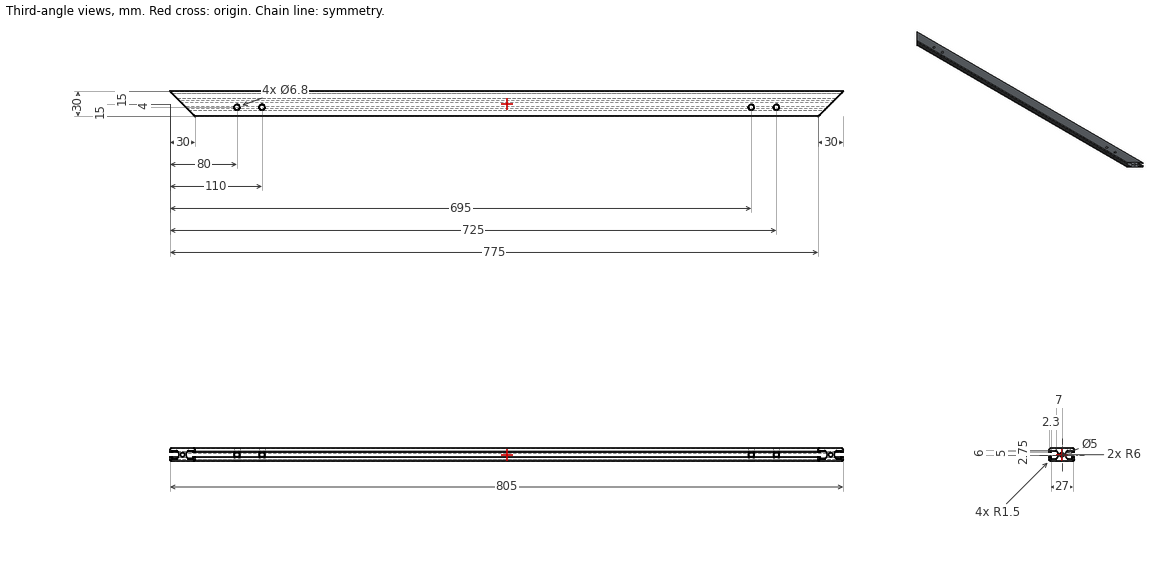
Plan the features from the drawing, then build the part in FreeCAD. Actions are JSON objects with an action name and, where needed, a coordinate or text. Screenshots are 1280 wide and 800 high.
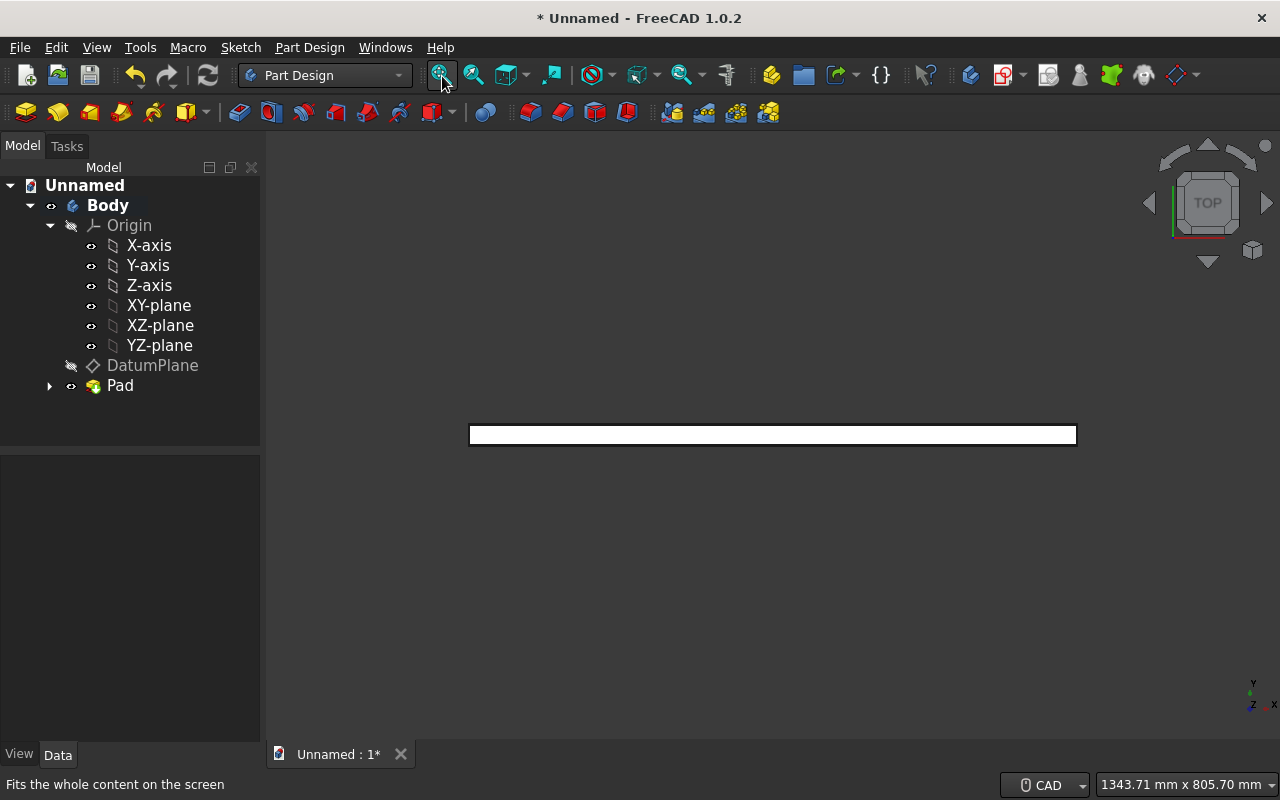
{"action": "left_click", "coordinate": [773, 434]}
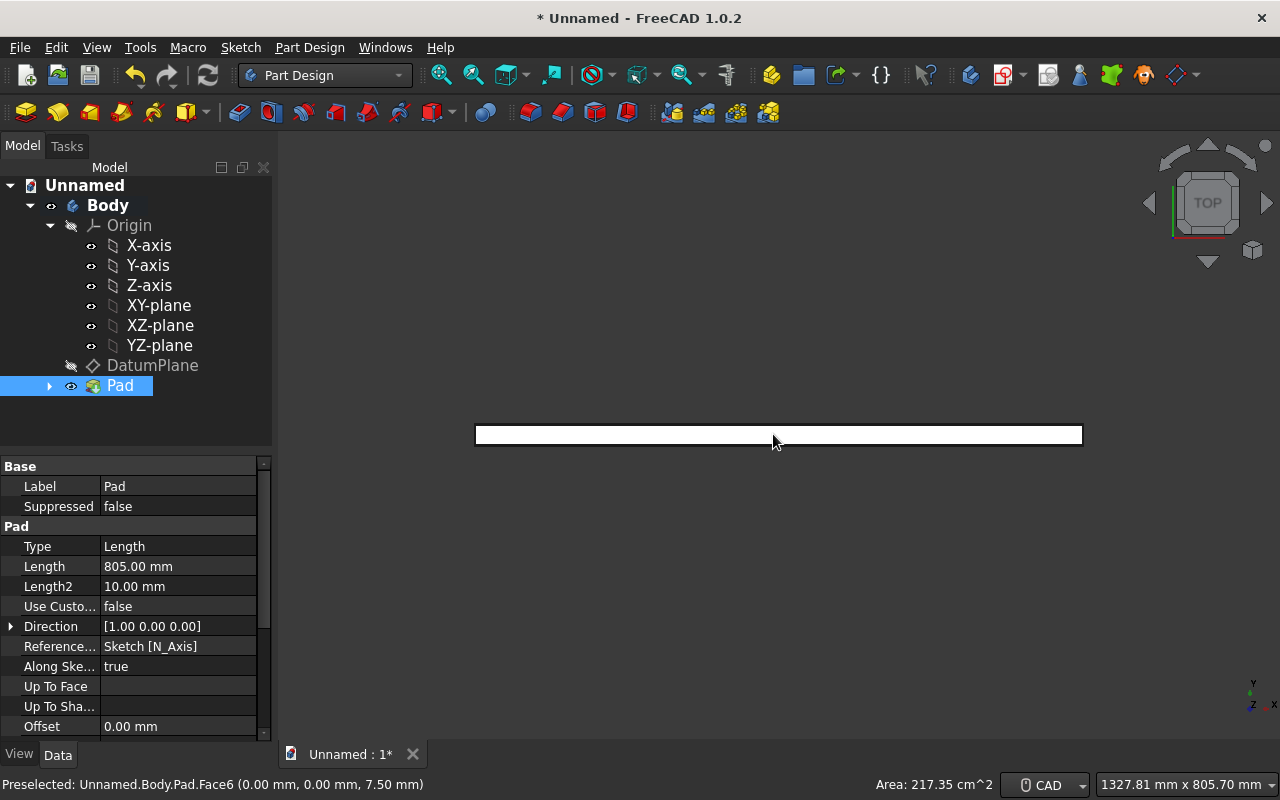
{"action": "left_click", "coordinate": [1004, 76]}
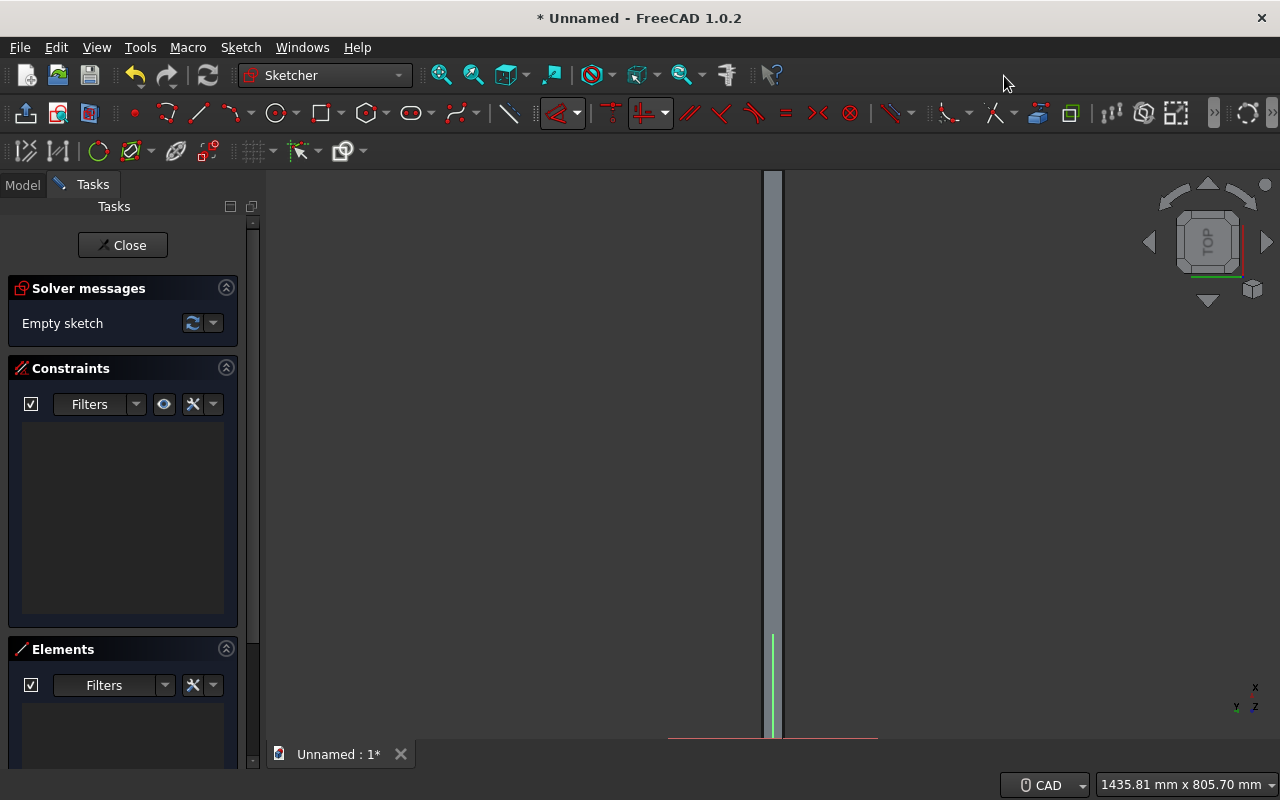
{"action": "scroll", "coordinate": [565, 455], "scroll_direction": "down", "scroll_amount": 2}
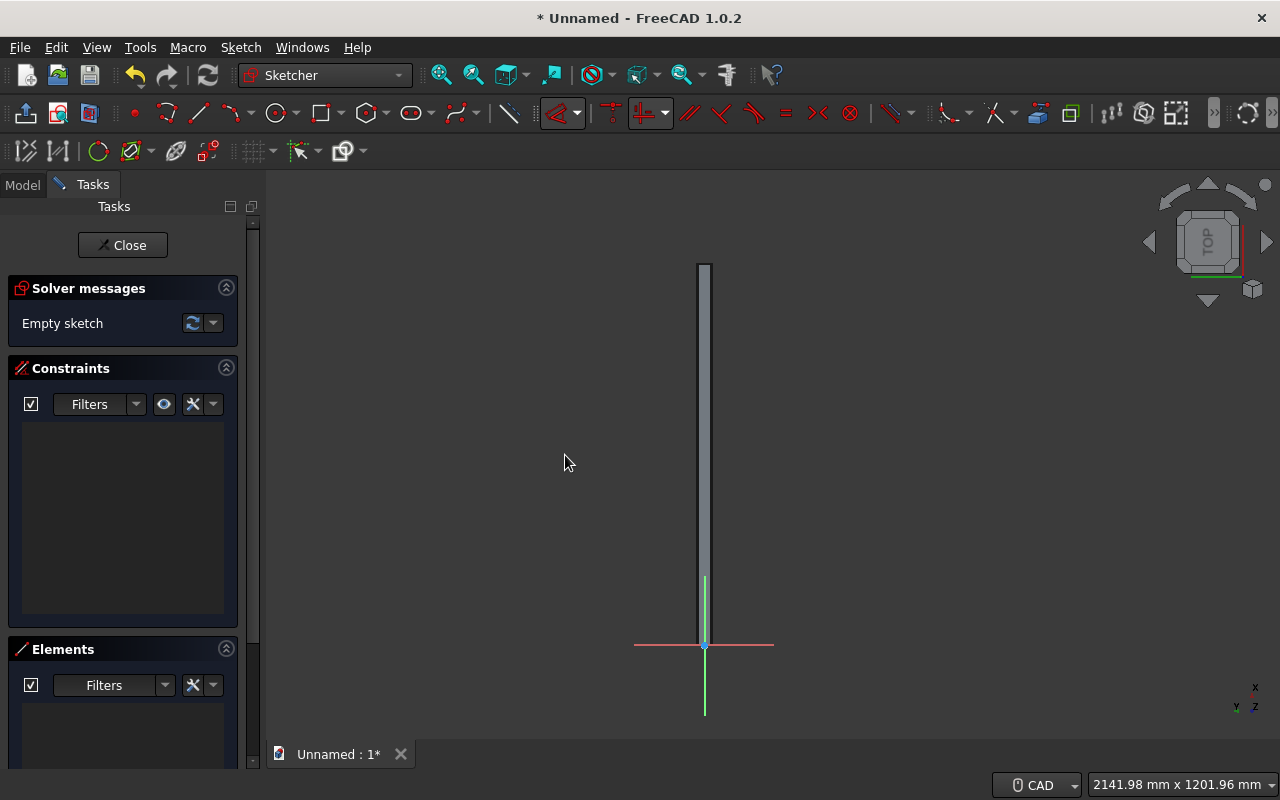
{"action": "left_click", "coordinate": [168, 114]}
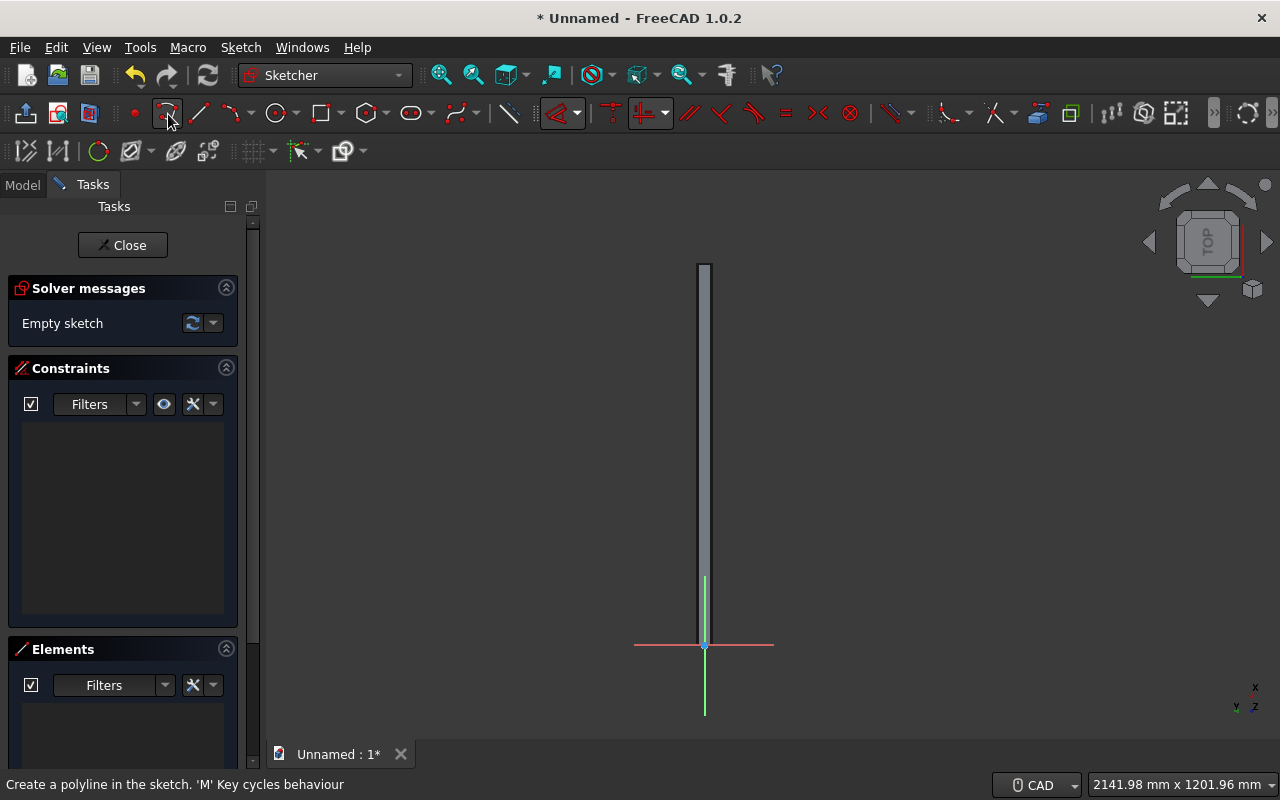
{"action": "scroll", "coordinate": [697, 645], "scroll_direction": "up", "scroll_amount": 5}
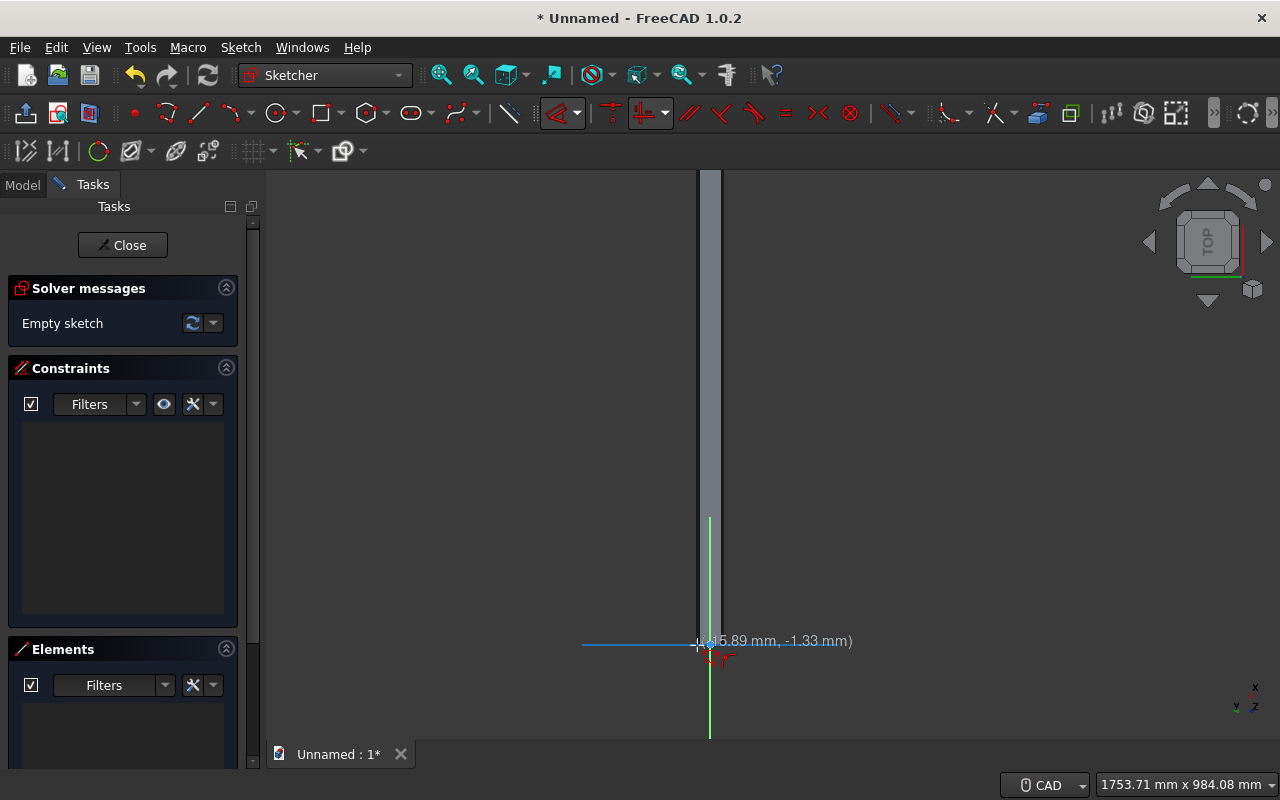
{"action": "left_click", "coordinate": [697, 645]}
{"action": "left_click", "coordinate": [736, 636]}
{"action": "left_click", "coordinate": [736, 606]}
{"action": "left_click", "coordinate": [697, 645]}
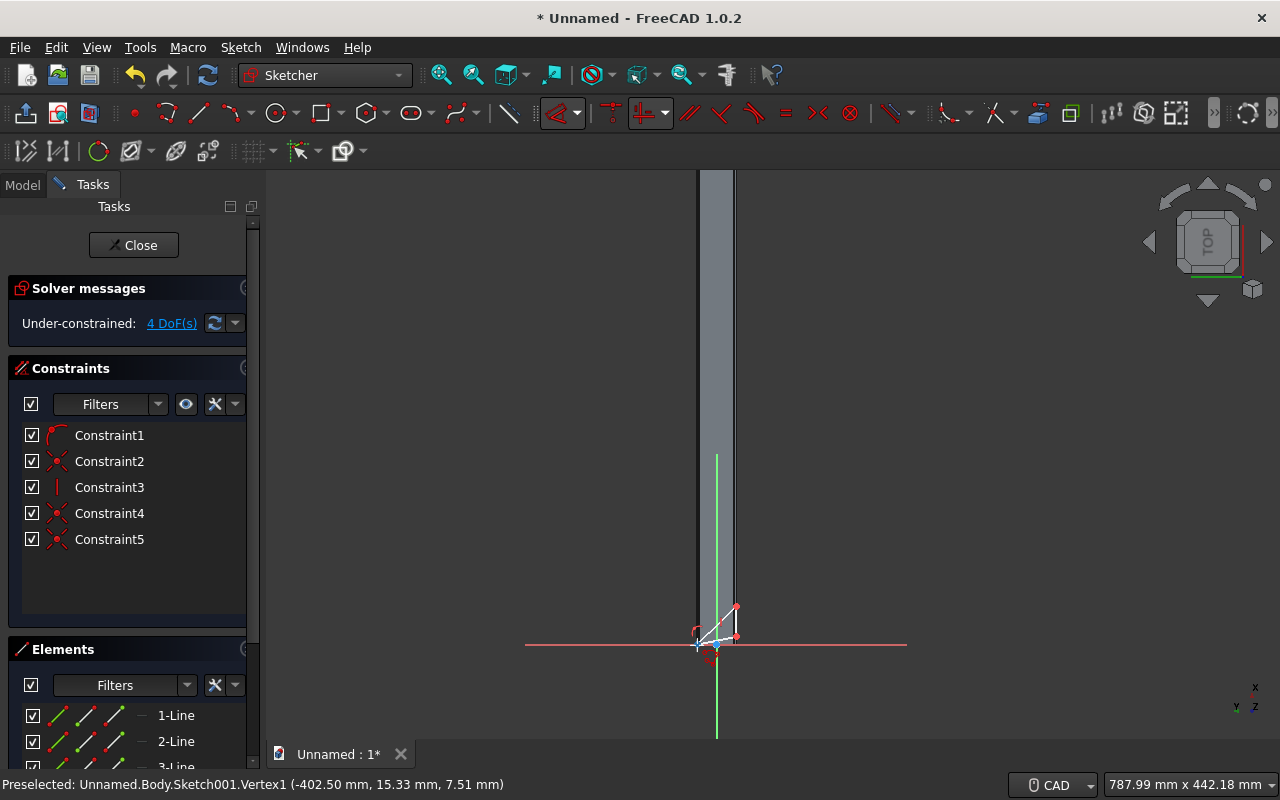
{"action": "scroll", "coordinate": [697, 645], "scroll_direction": "down", "scroll_amount": 5}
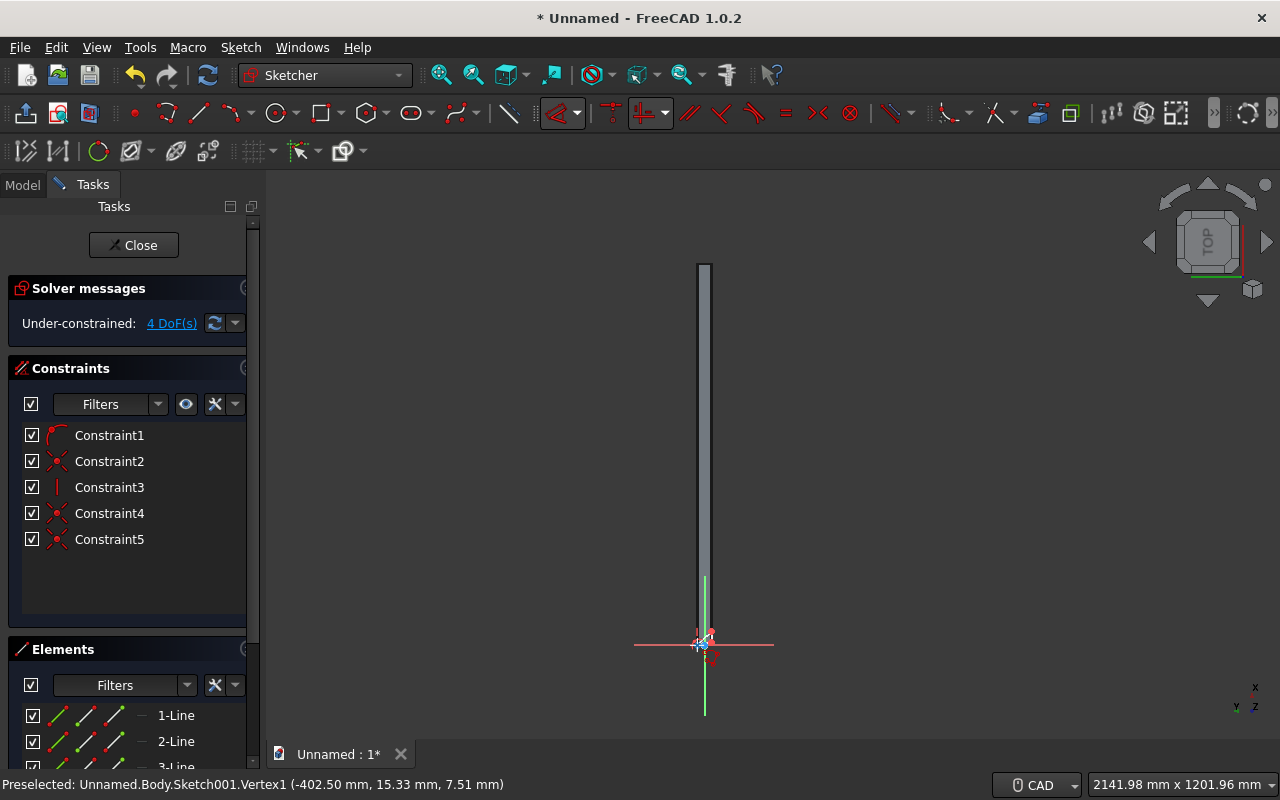
{"action": "scroll", "coordinate": [712, 278], "scroll_direction": "up", "scroll_amount": 5}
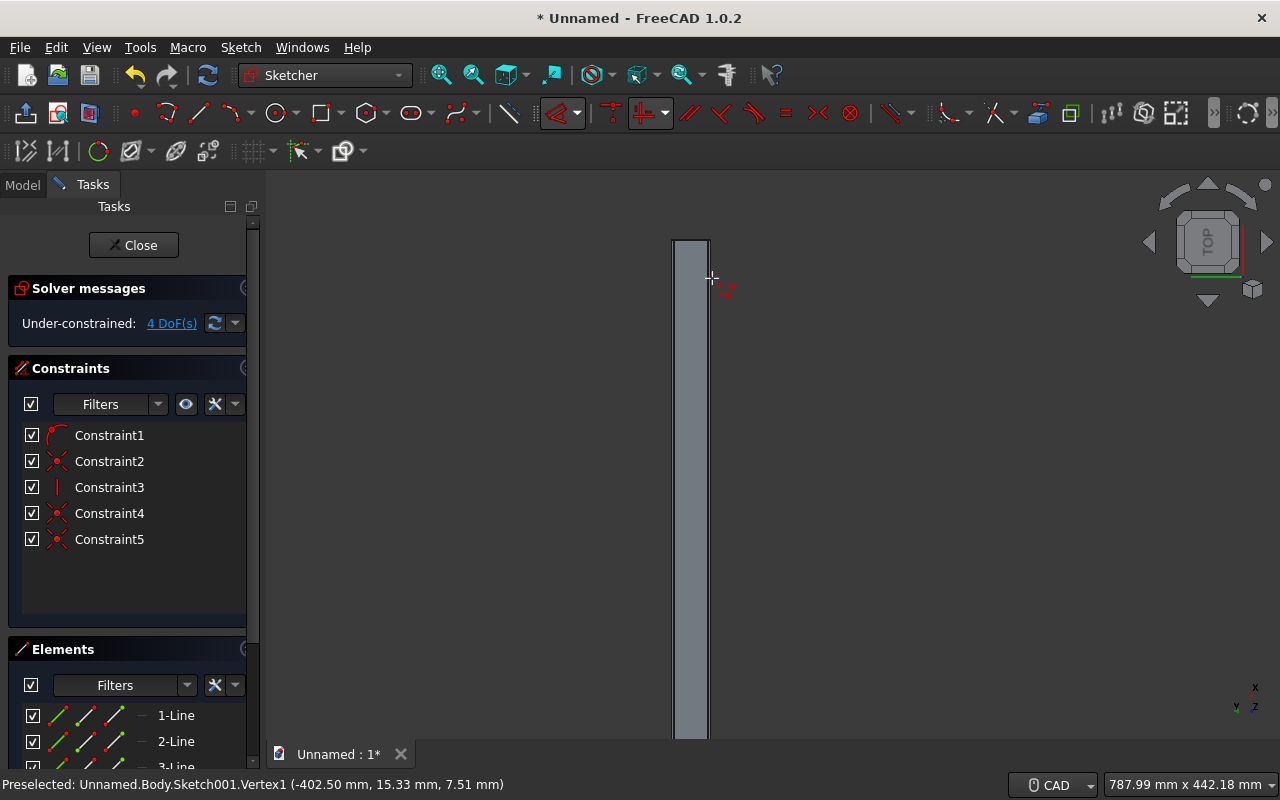
{"action": "left_click", "coordinate": [710, 279]}
{"action": "left_click", "coordinate": [710, 240]}
{"action": "left_click", "coordinate": [672, 240]}
{"action": "left_click", "coordinate": [710, 280]}
{"action": "key", "text": "Escape"}
{"action": "key", "text": "Escape"}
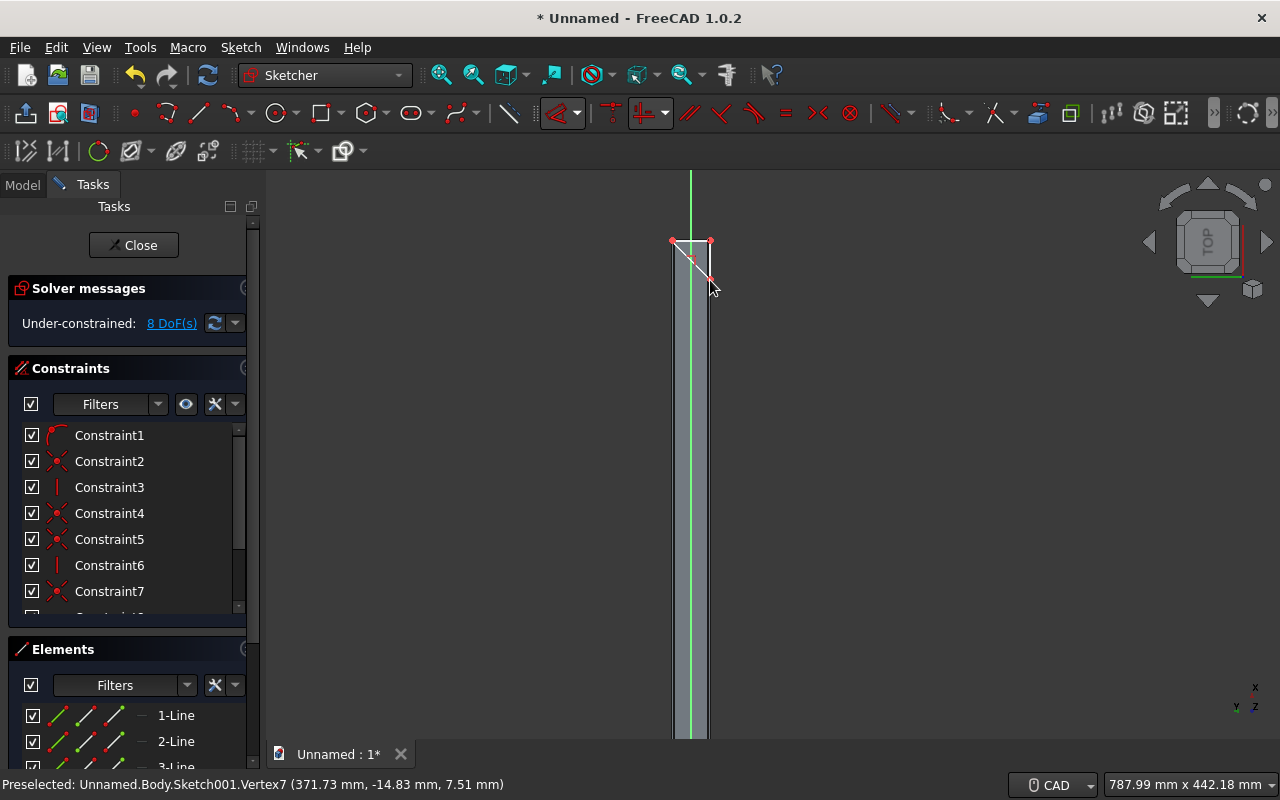
{"action": "scroll", "coordinate": [712, 278], "scroll_direction": "down", "scroll_amount": 5}